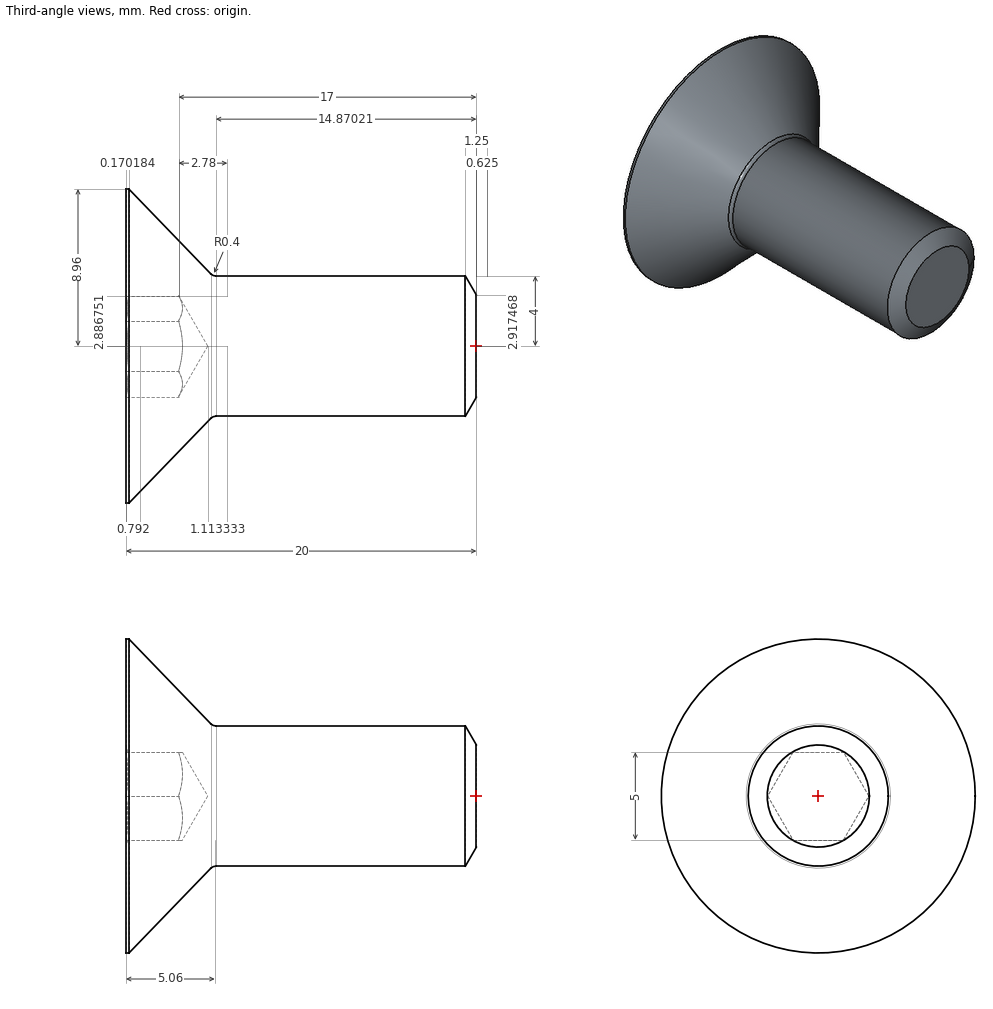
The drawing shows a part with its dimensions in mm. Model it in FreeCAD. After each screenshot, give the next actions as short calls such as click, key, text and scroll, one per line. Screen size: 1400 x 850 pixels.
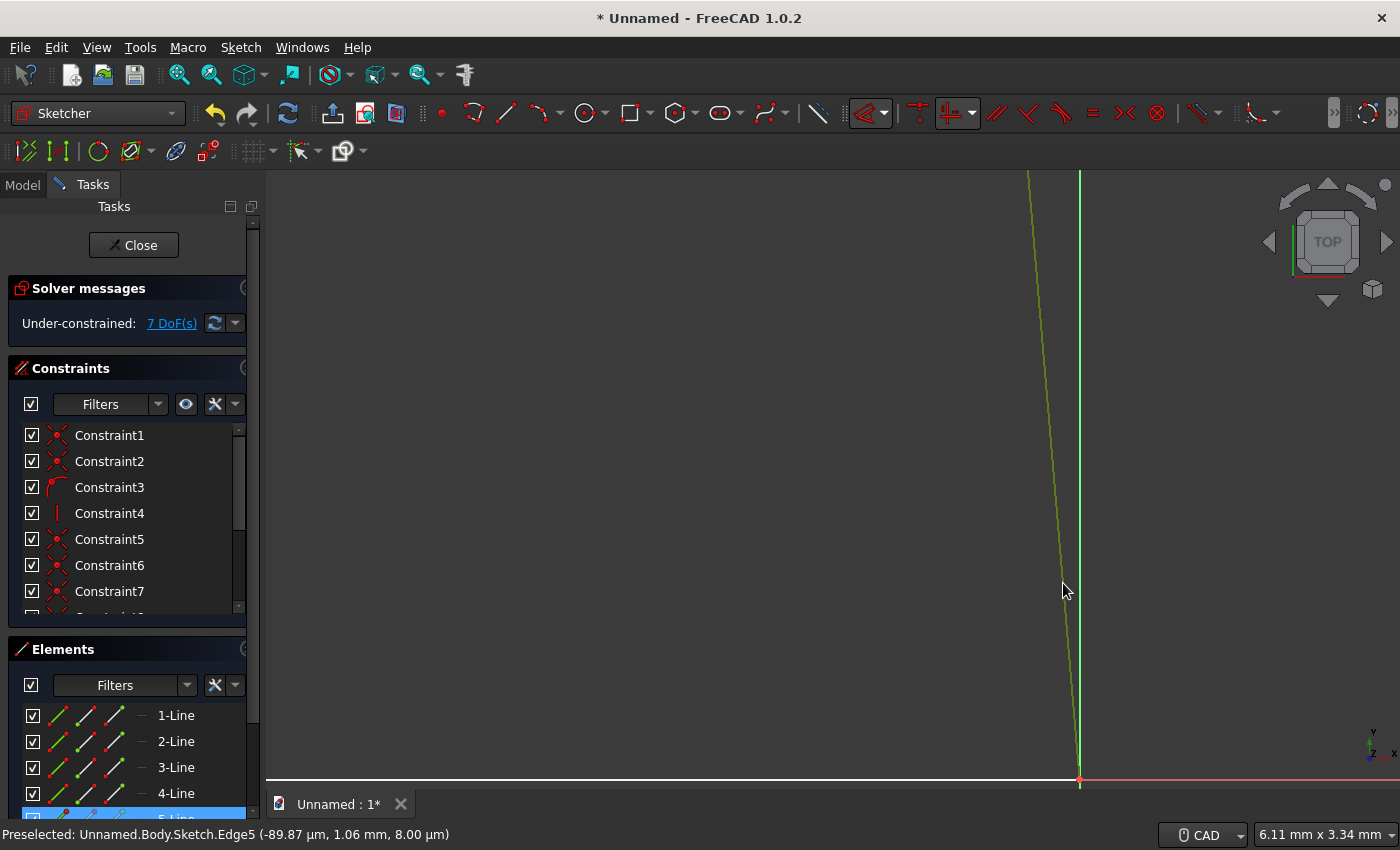
click(974, 114)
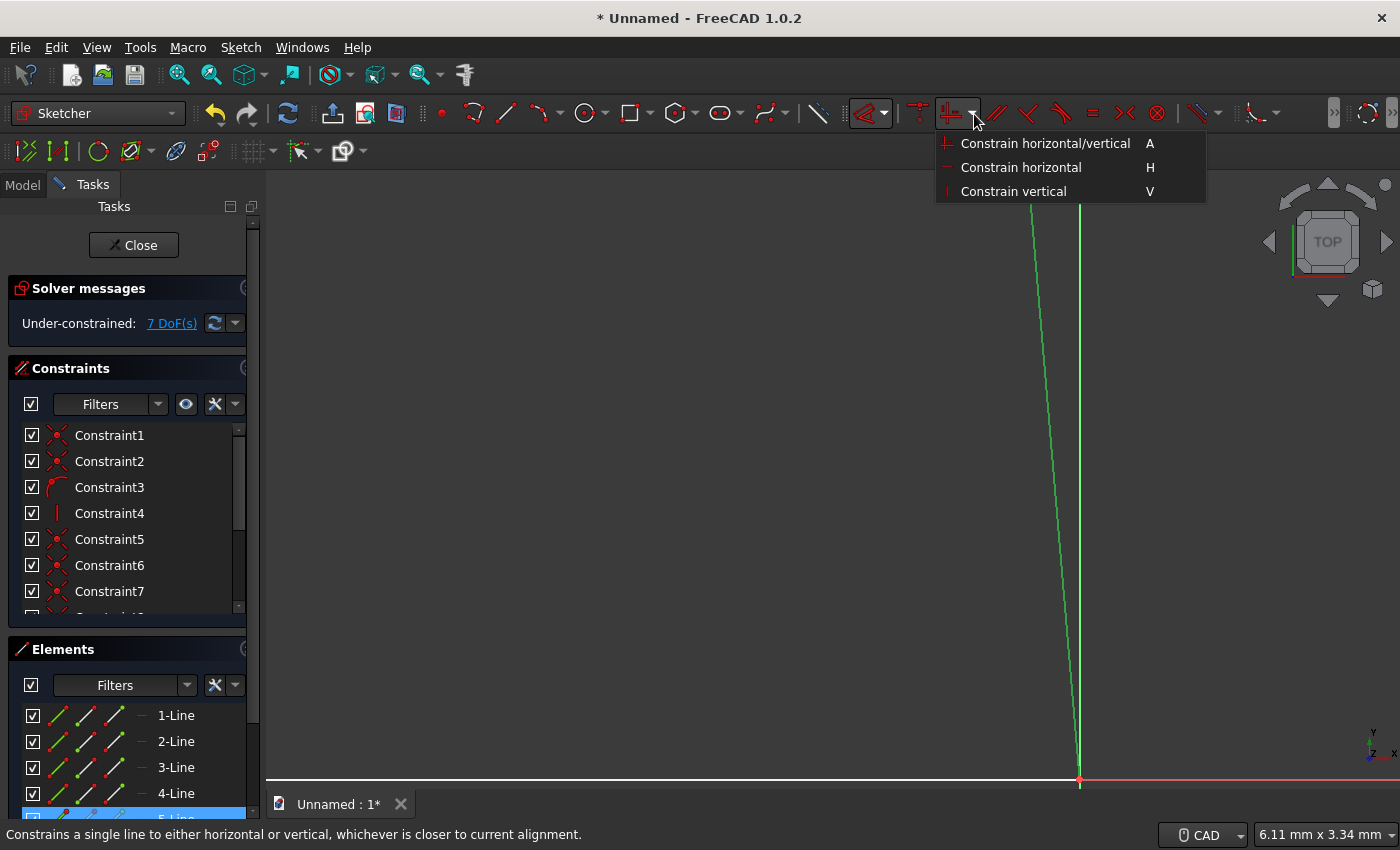
click(1071, 191)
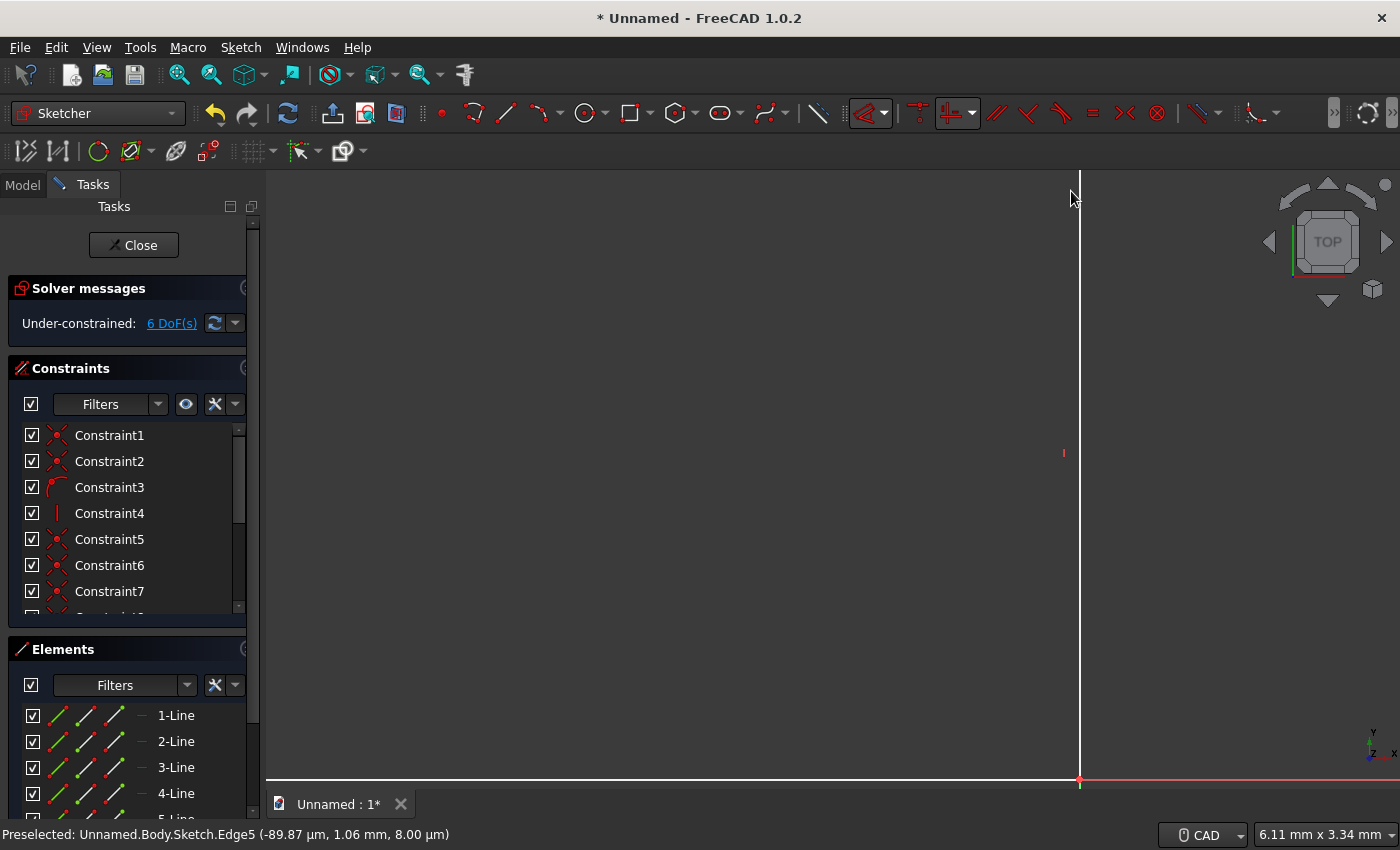
click(864, 114)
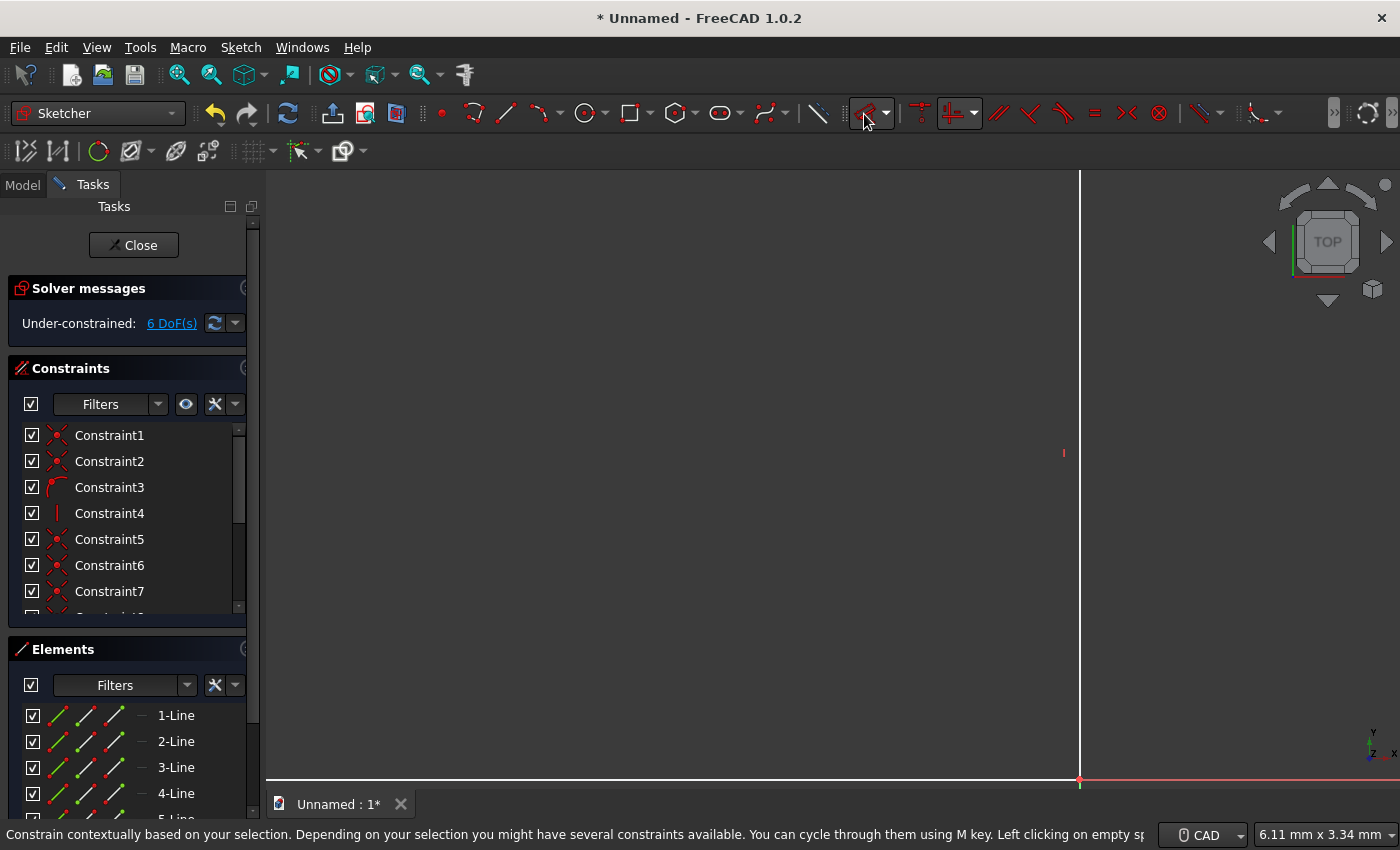
scroll(1069, 585, down, 9)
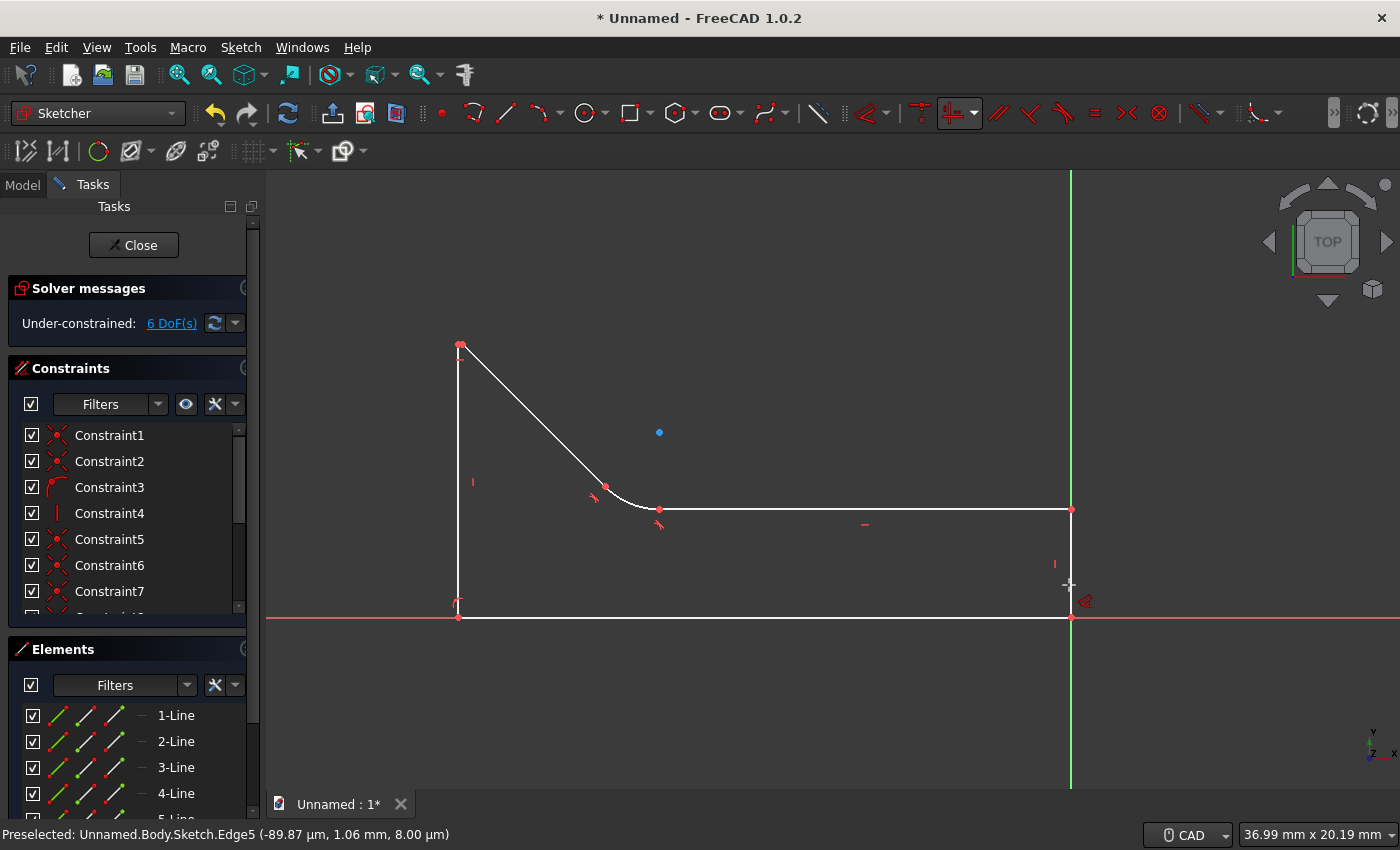
scroll(620, 498, up, 6)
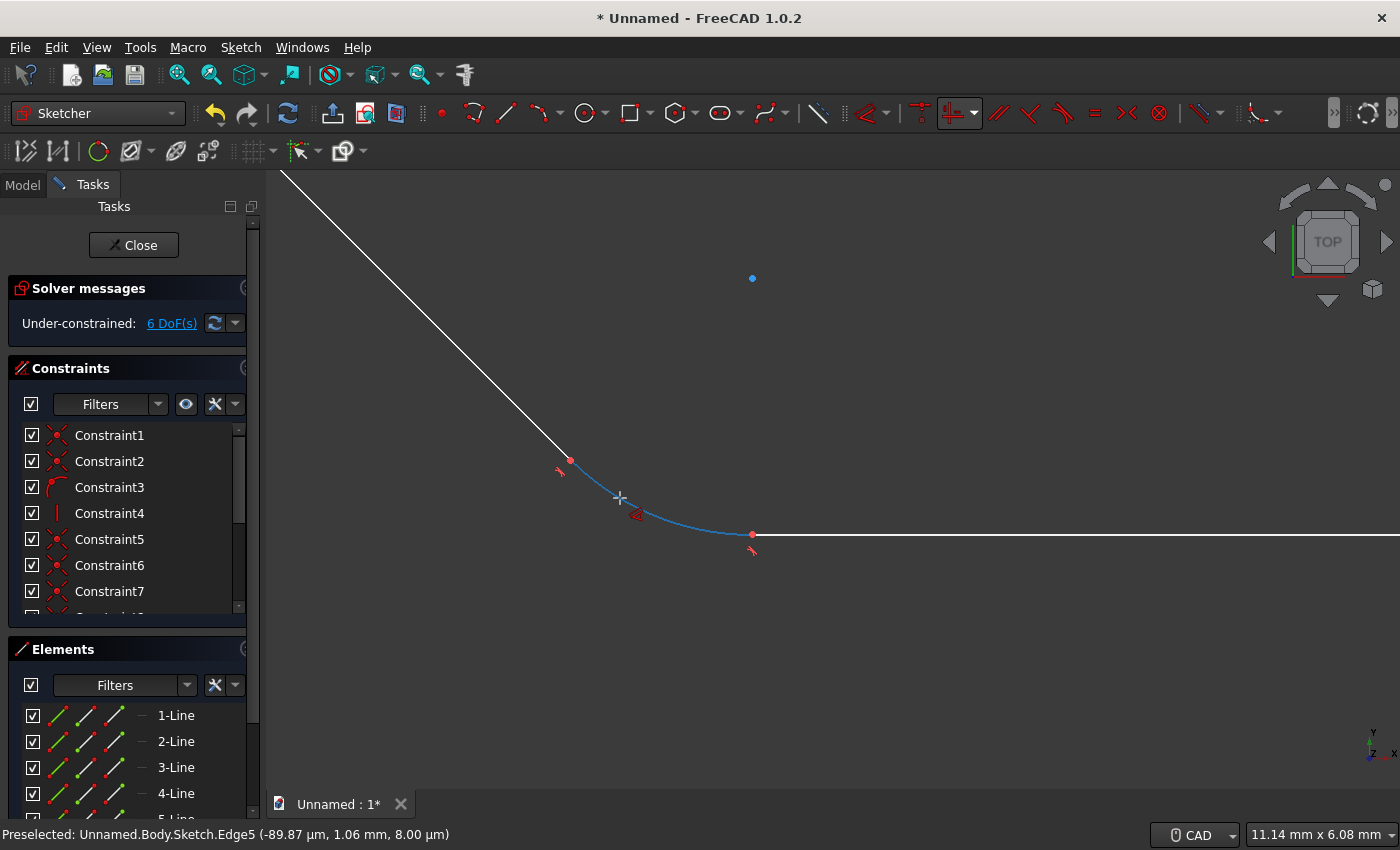
click(618, 497)
click(601, 524)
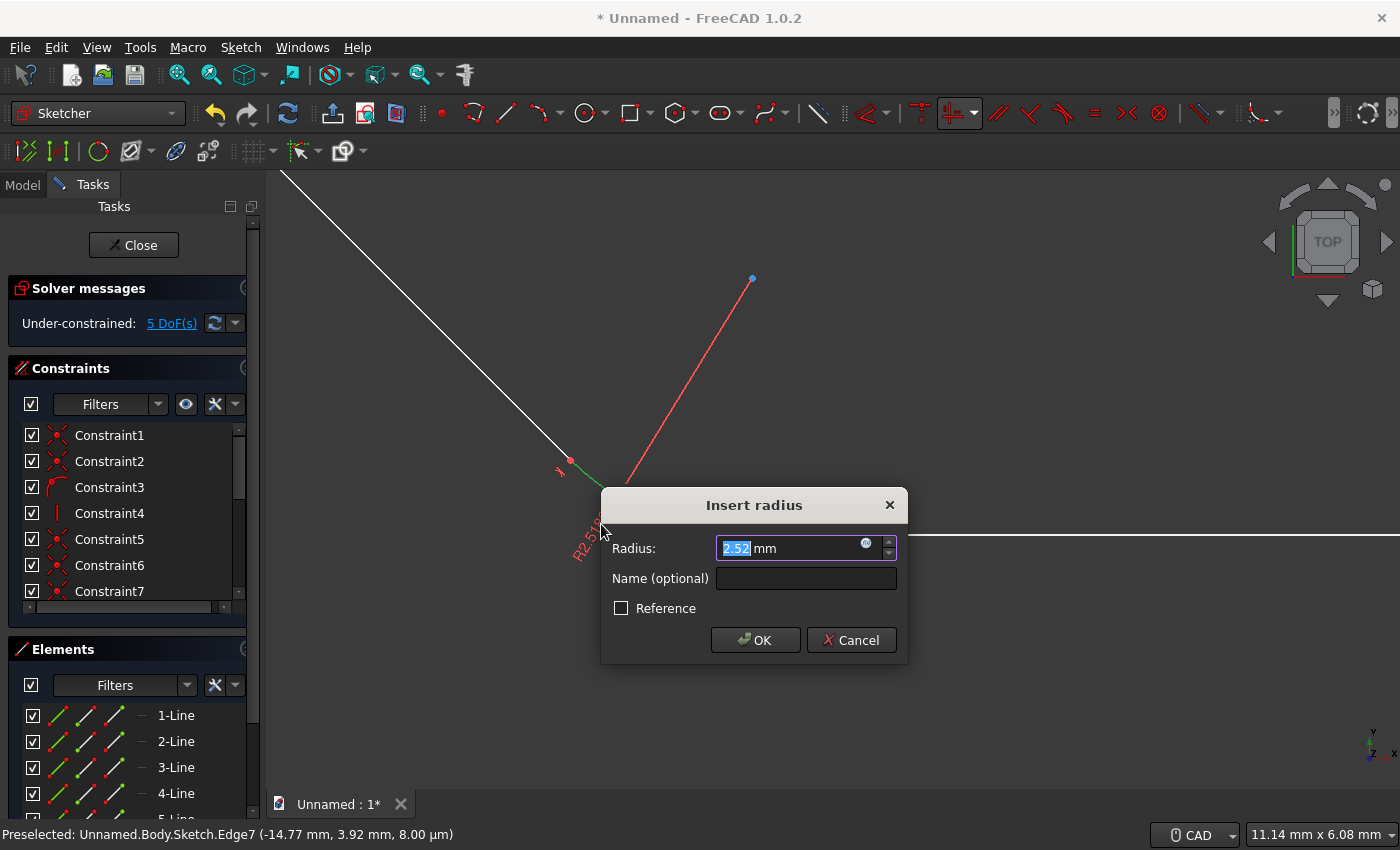
text(0.4)
key(Return)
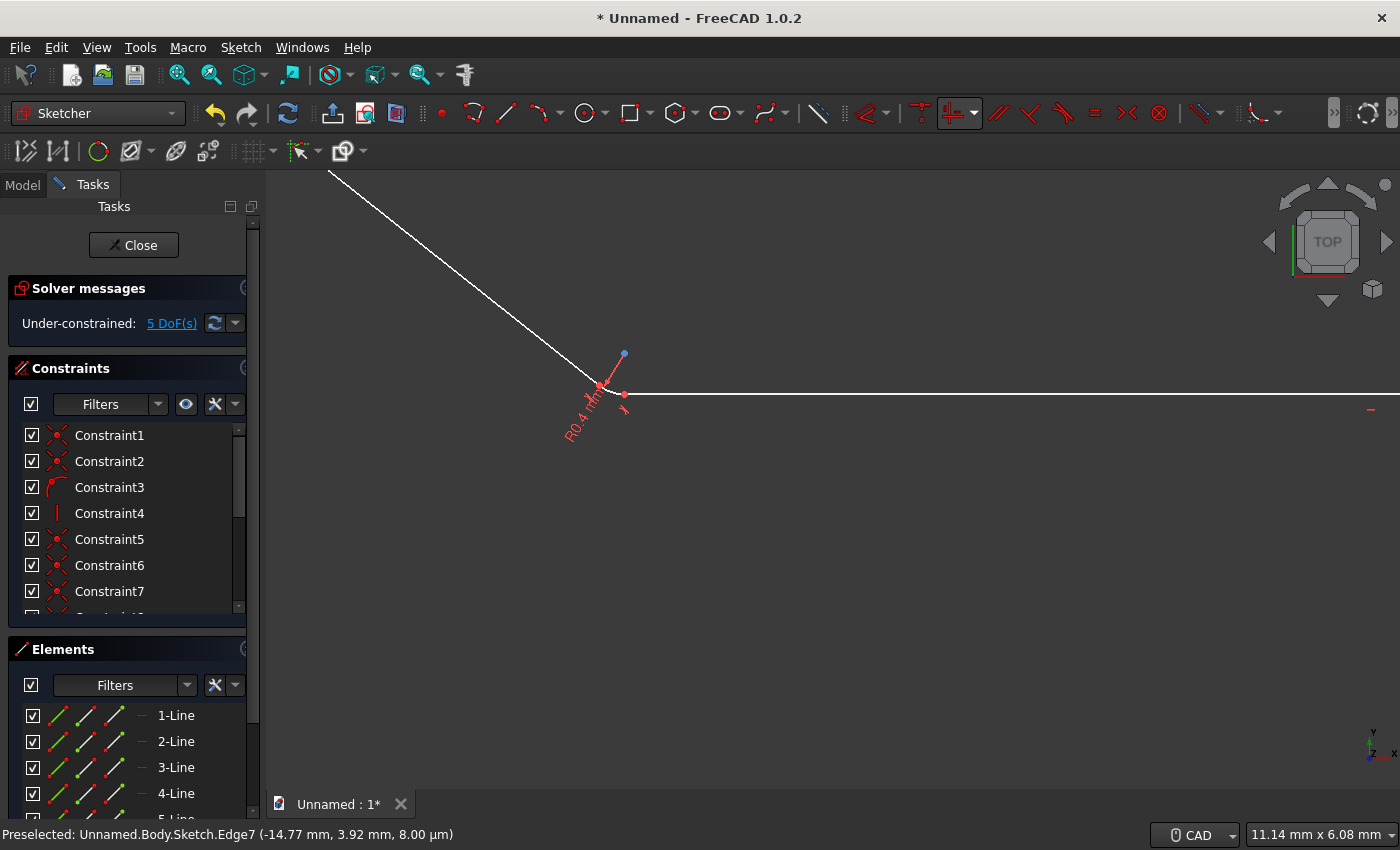
scroll(620, 497, down, 6)